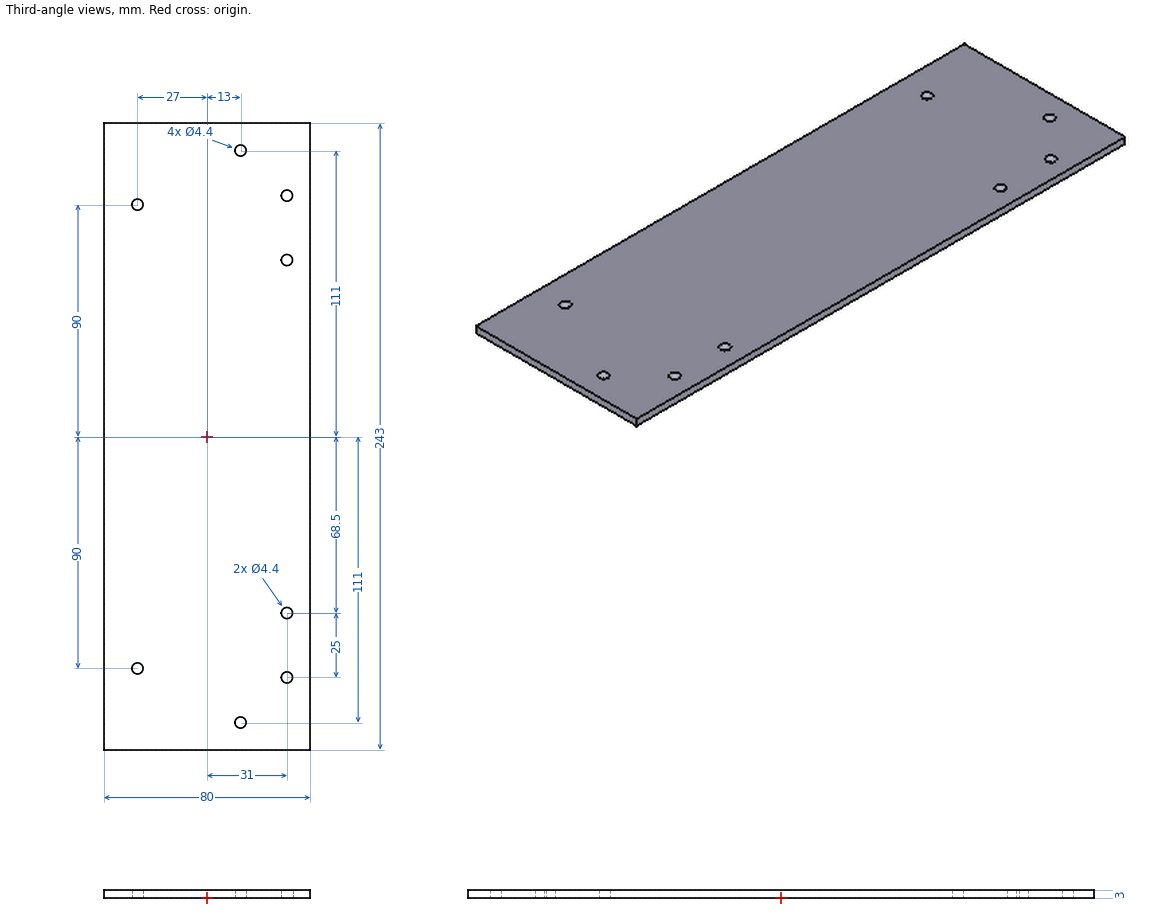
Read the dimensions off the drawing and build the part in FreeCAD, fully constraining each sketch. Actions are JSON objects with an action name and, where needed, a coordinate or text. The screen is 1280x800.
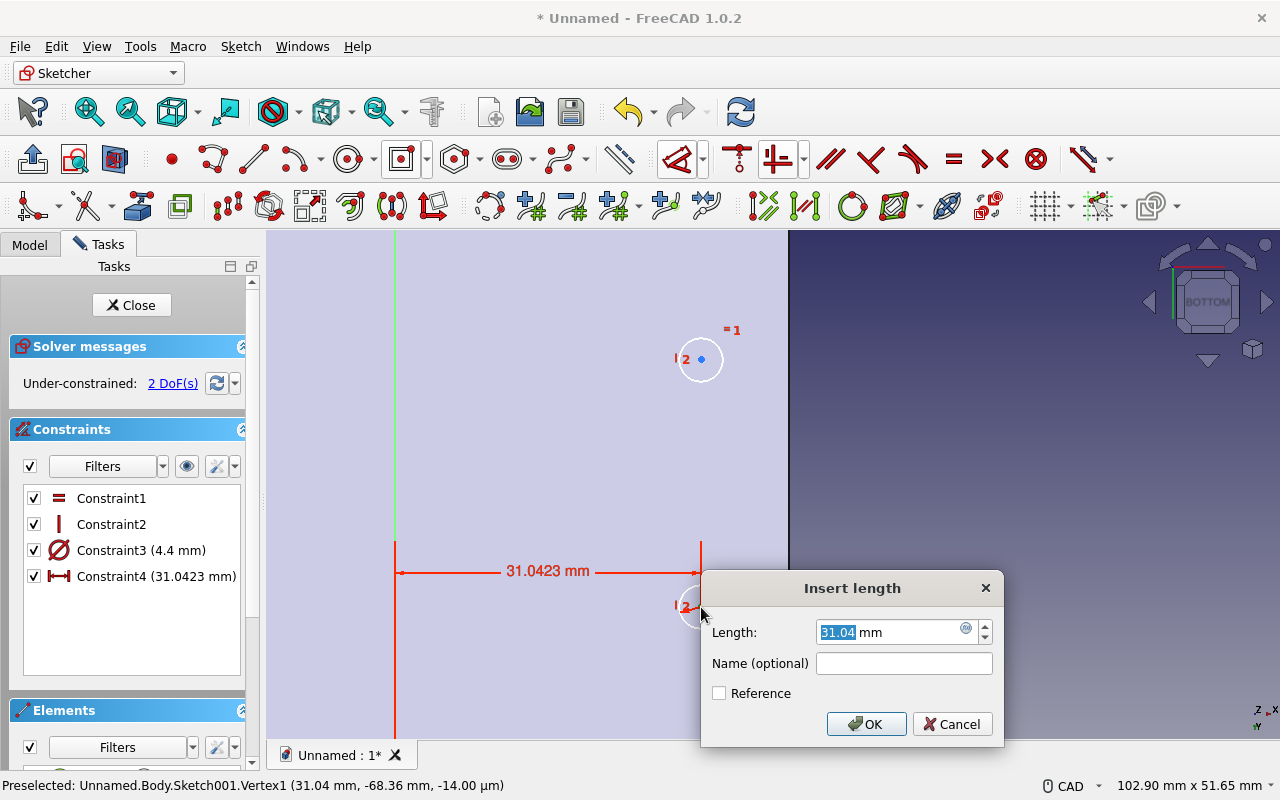
{"action": "type", "text": "31"}
{"action": "key", "text": "Return"}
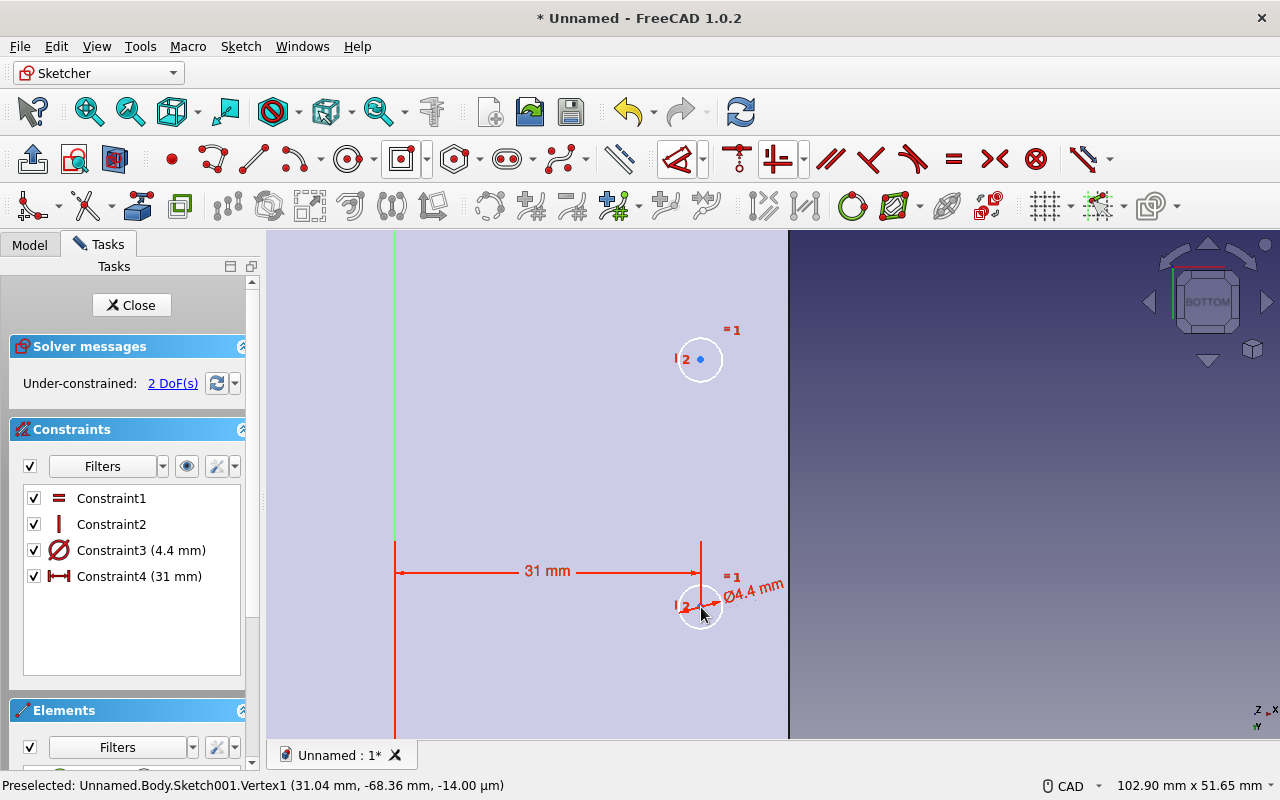
{"action": "left_click", "coordinate": [701, 607]}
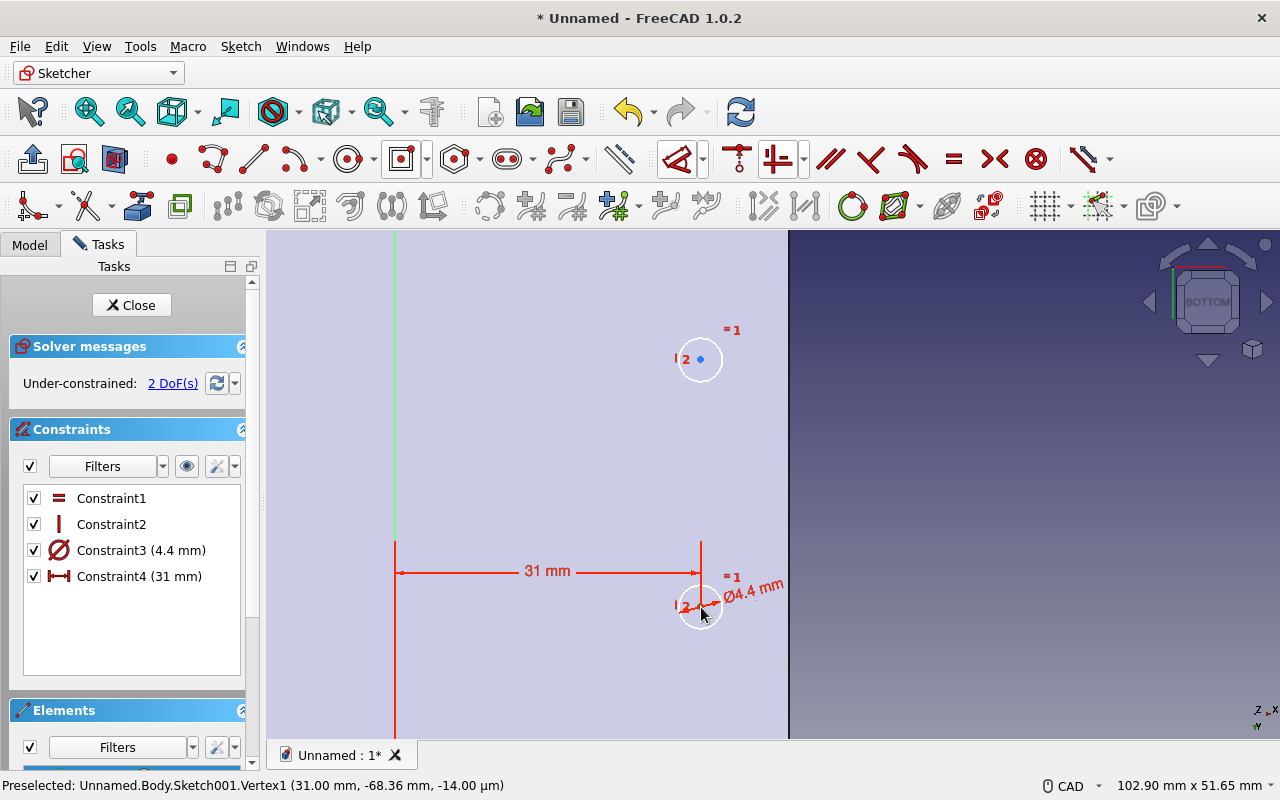
{"action": "left_click", "coordinate": [701, 360]}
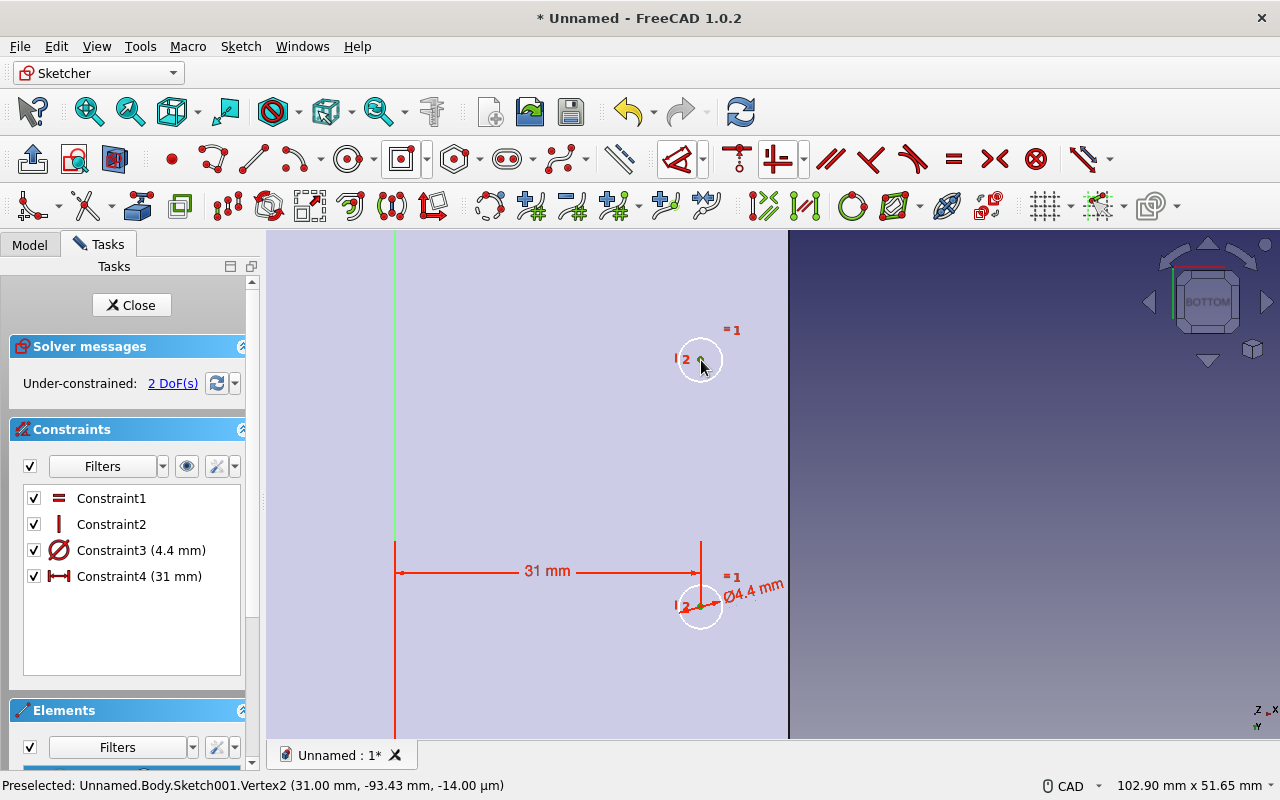
{"action": "left_click", "coordinate": [702, 160]}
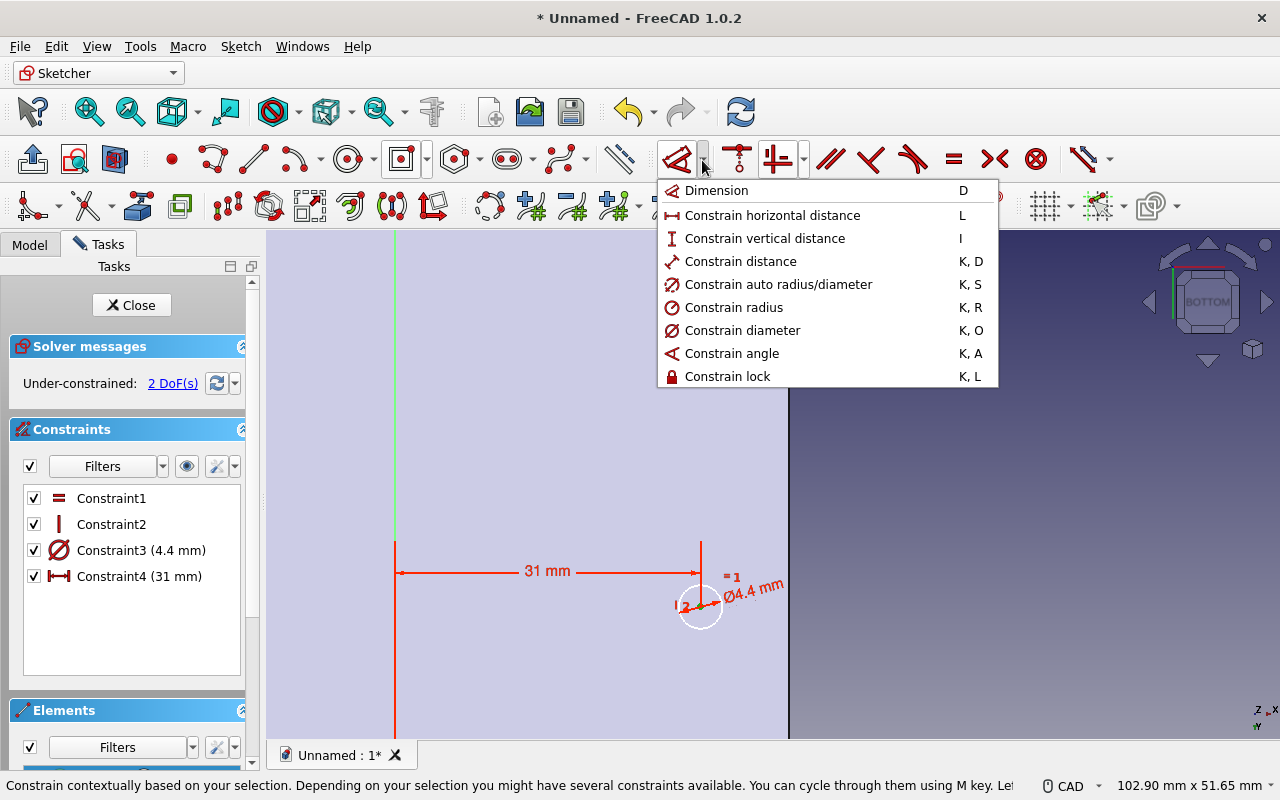
{"action": "left_click", "coordinate": [828, 238]}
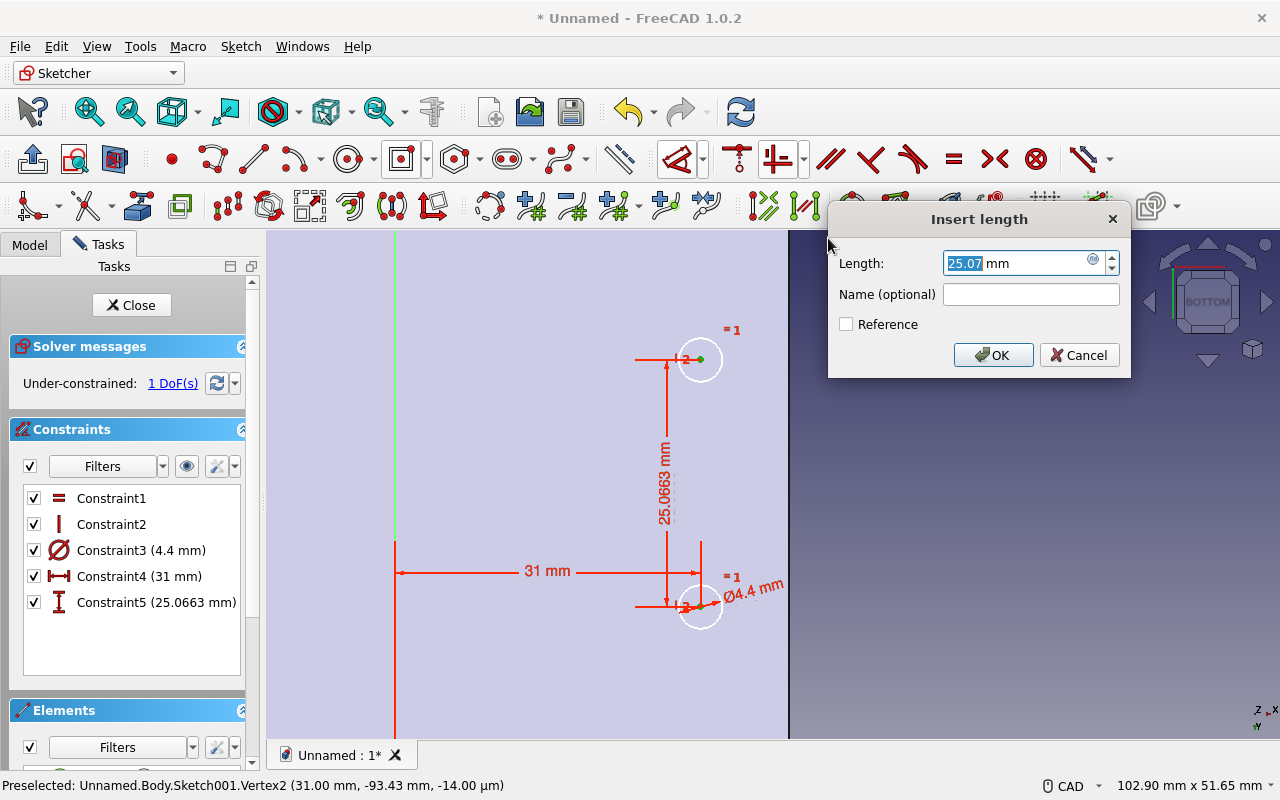
{"action": "type", "text": "25"}
{"action": "key", "text": "Return"}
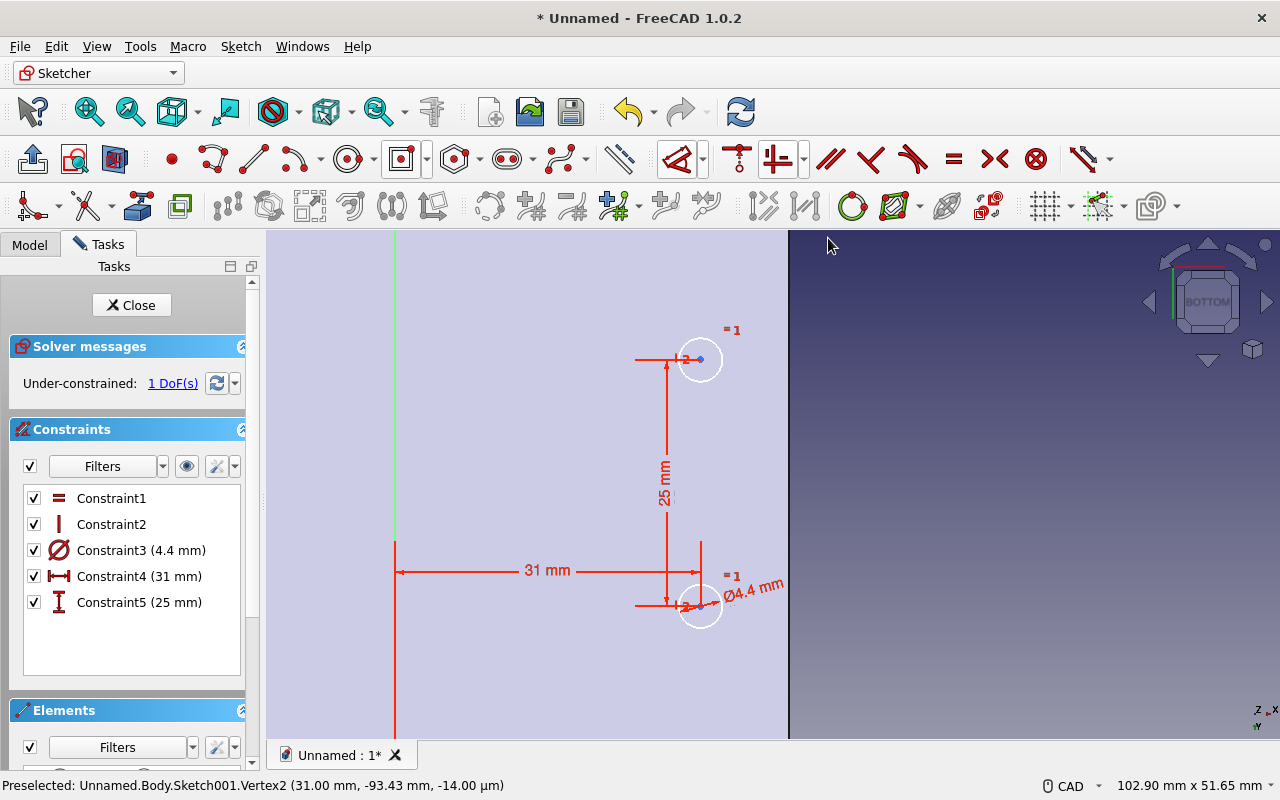
{"action": "left_click", "coordinate": [701, 606]}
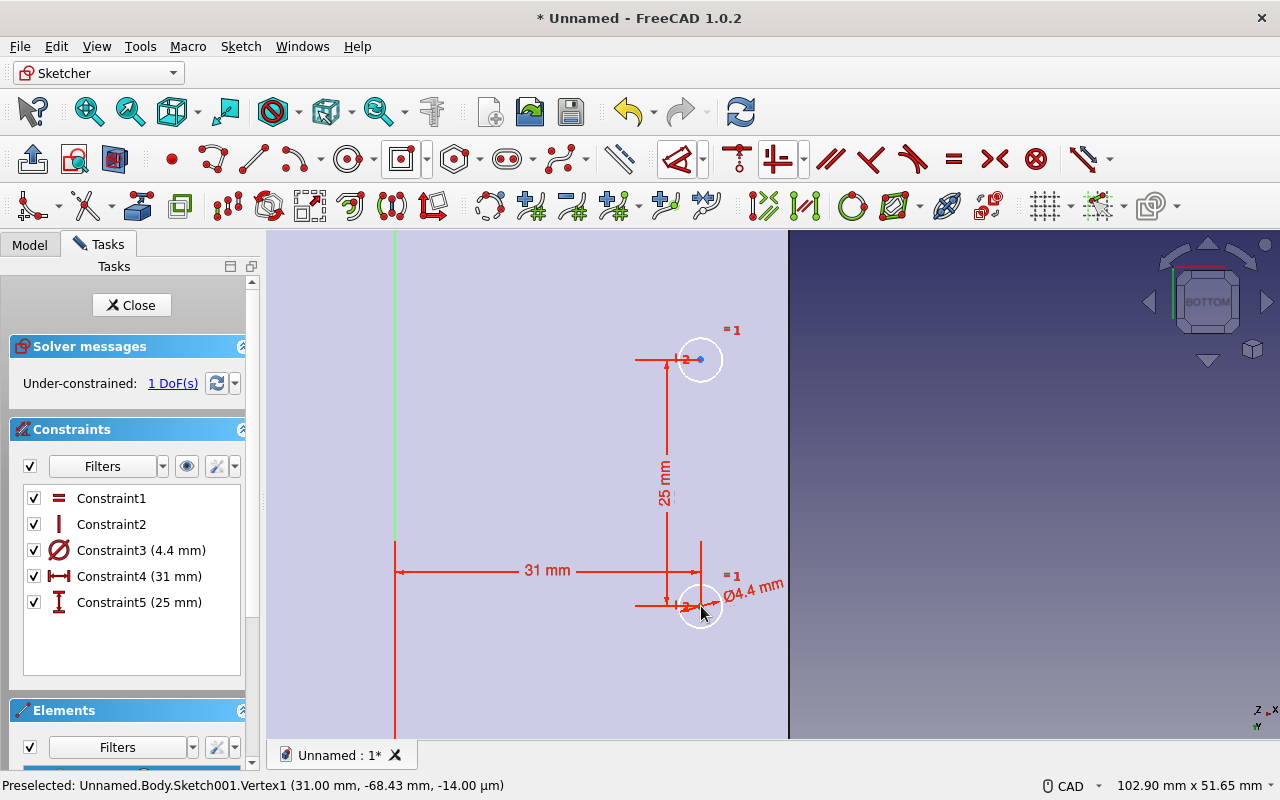
{"action": "left_click", "coordinate": [702, 160]}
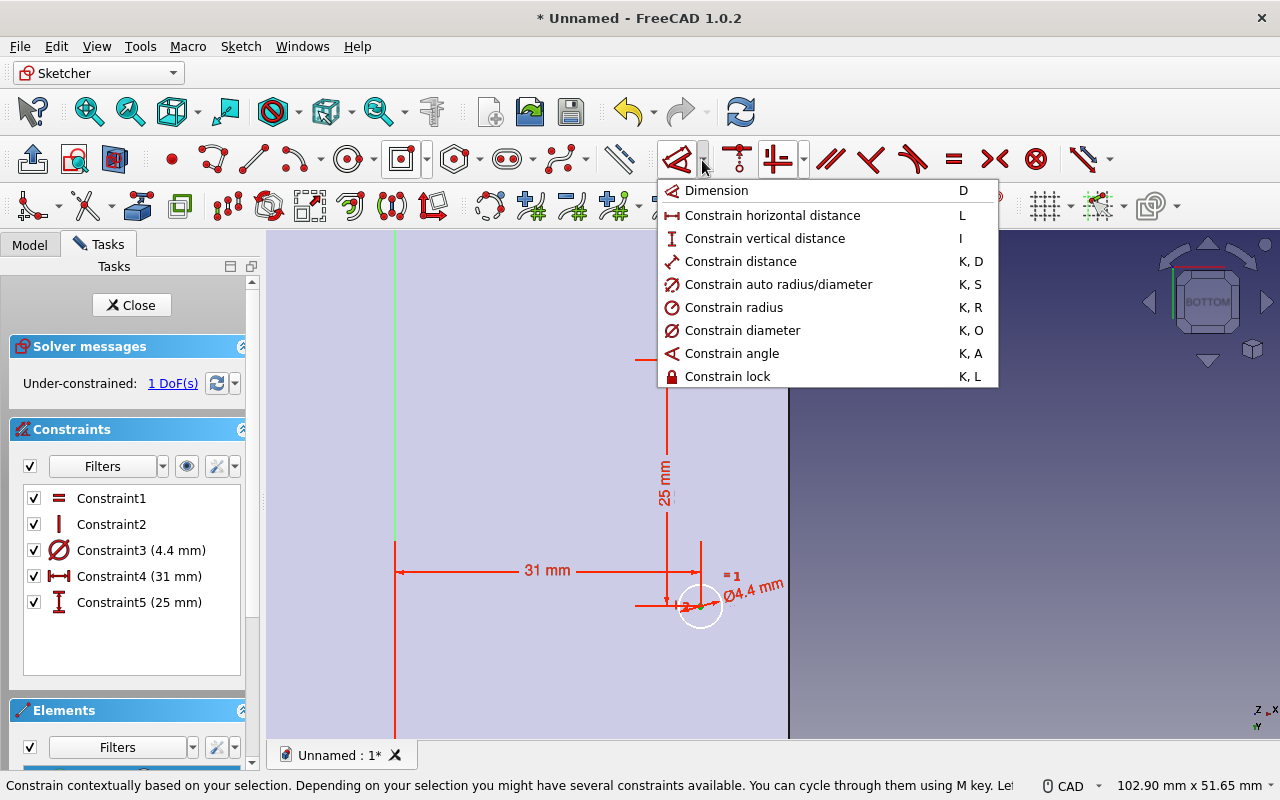
{"action": "left_click", "coordinate": [828, 238]}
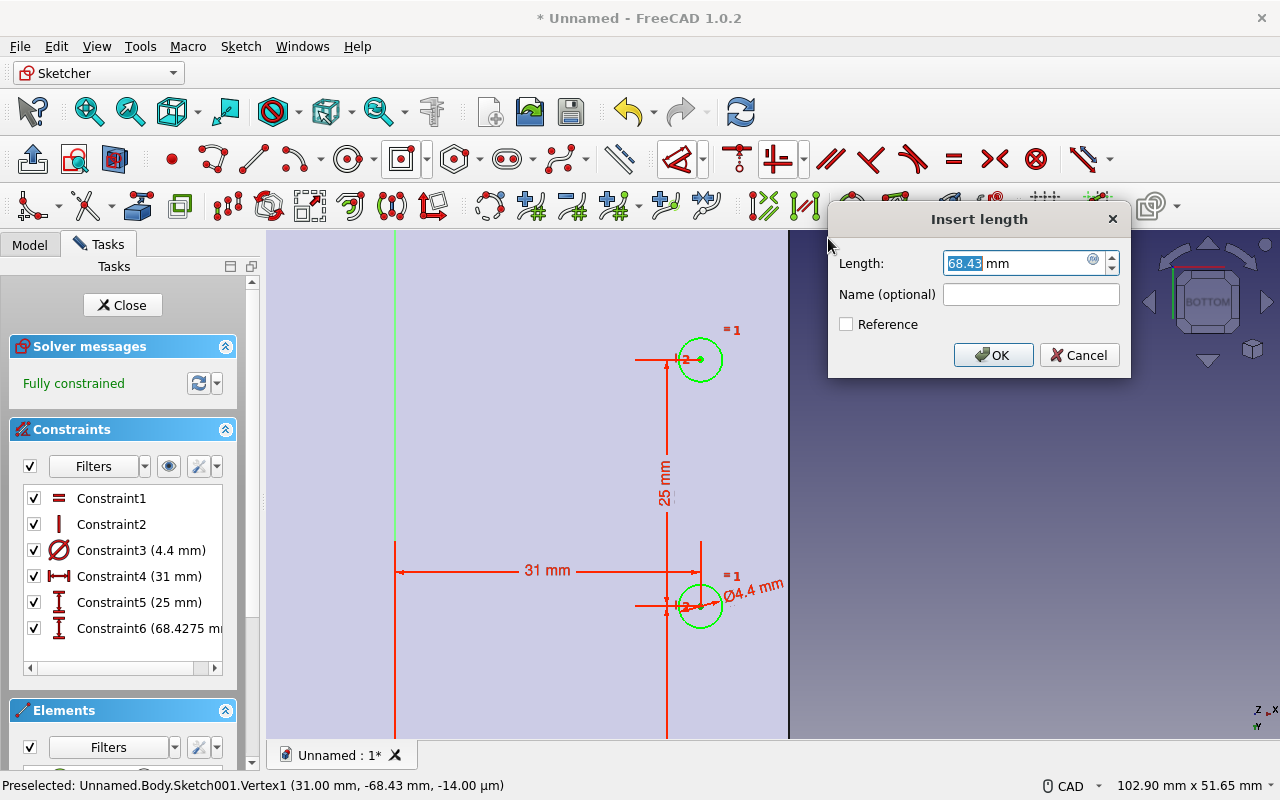
{"action": "type", "text": "68.5"}
{"action": "key", "text": "Return"}